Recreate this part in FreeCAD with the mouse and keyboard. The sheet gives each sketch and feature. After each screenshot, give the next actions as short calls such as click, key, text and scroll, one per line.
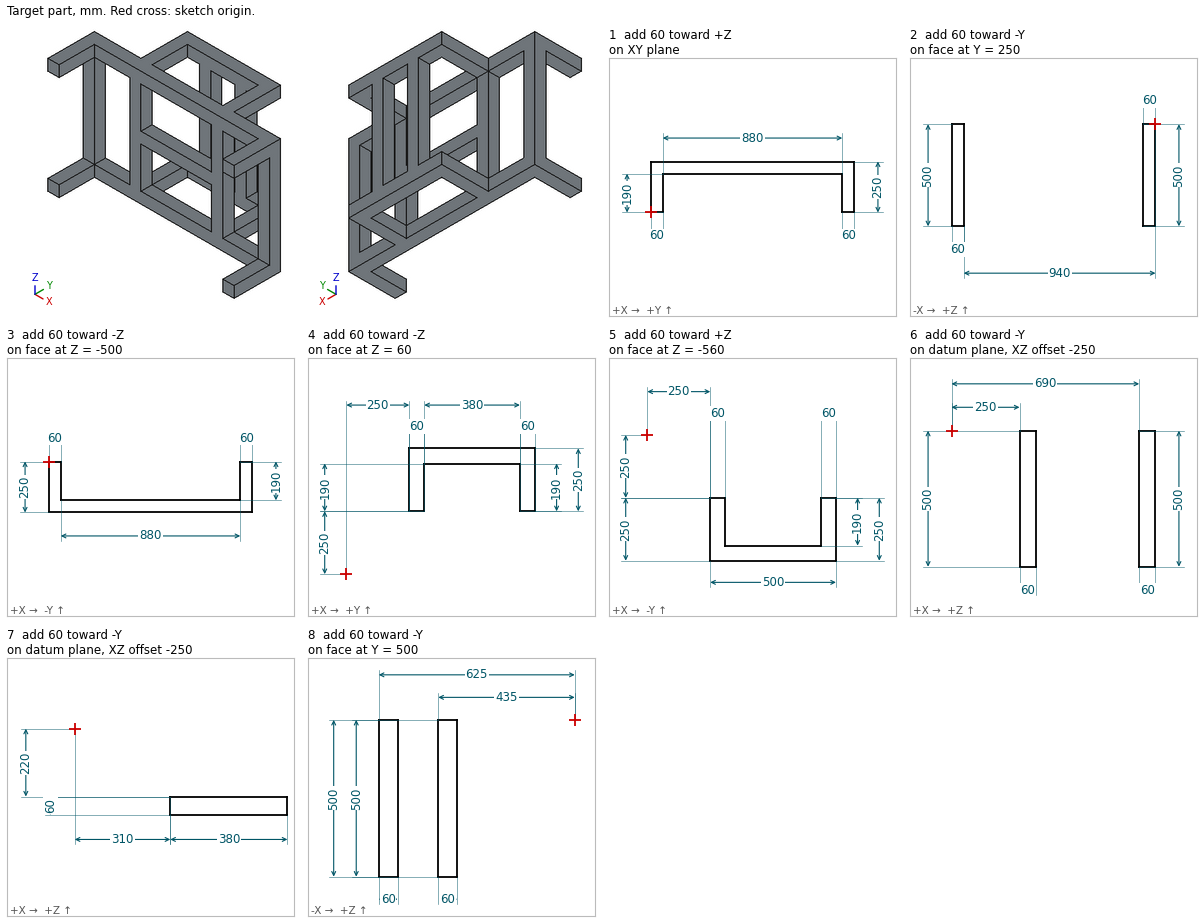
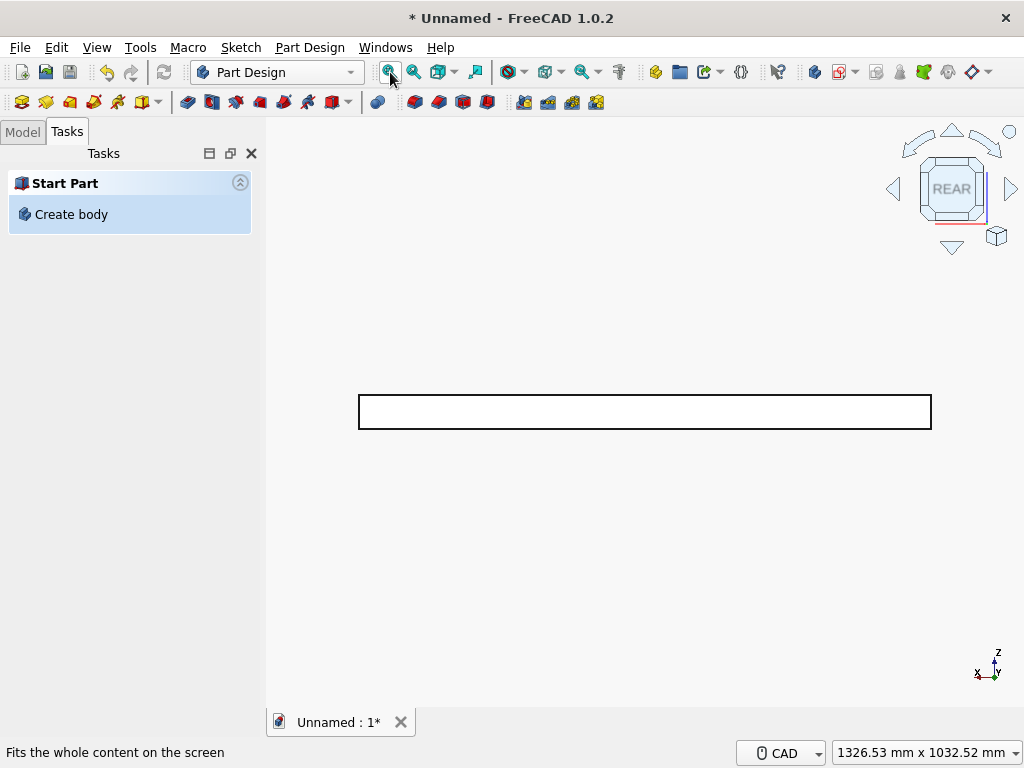
click(400, 411)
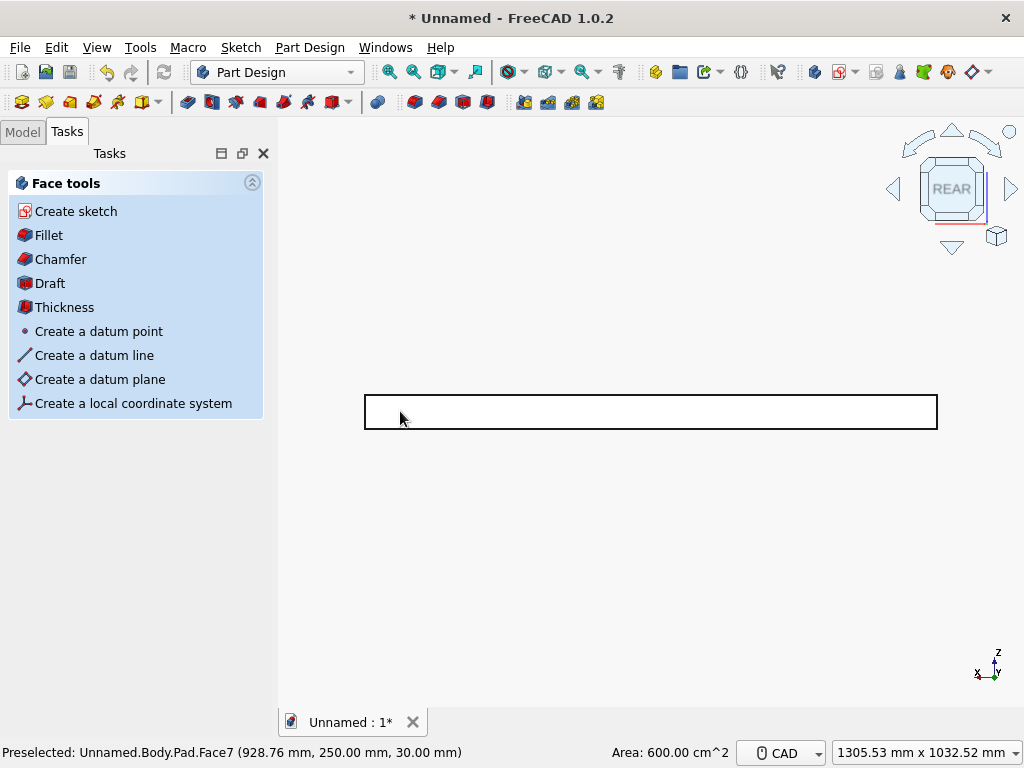
click(840, 72)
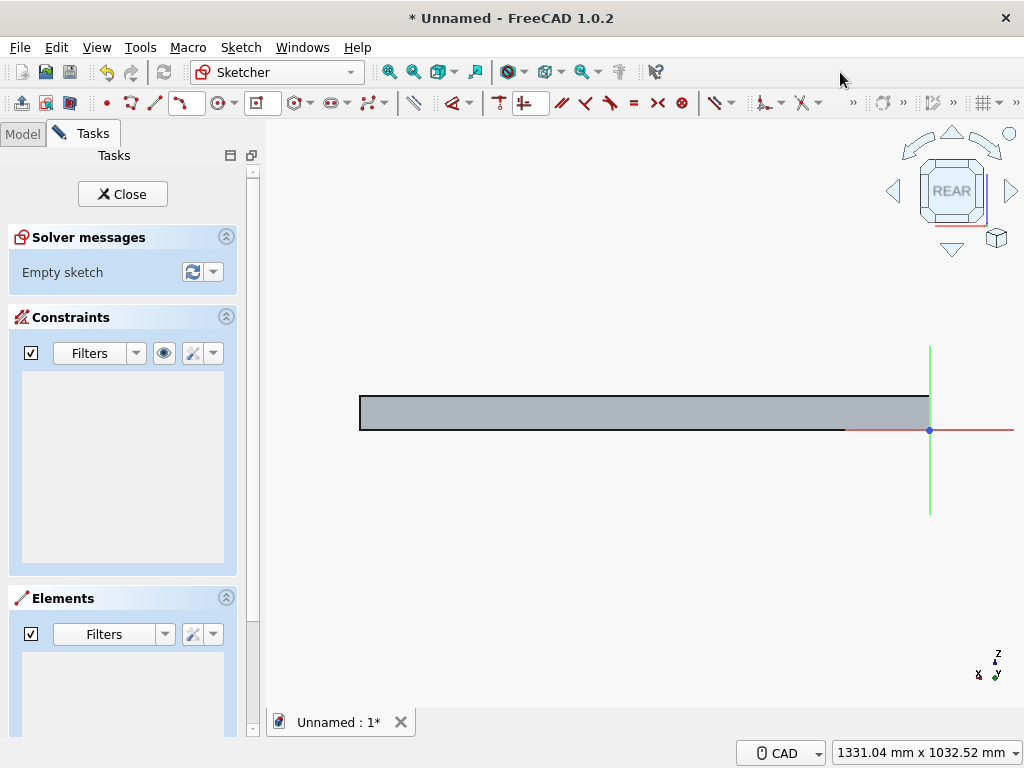
scroll(437, 147, down, 2)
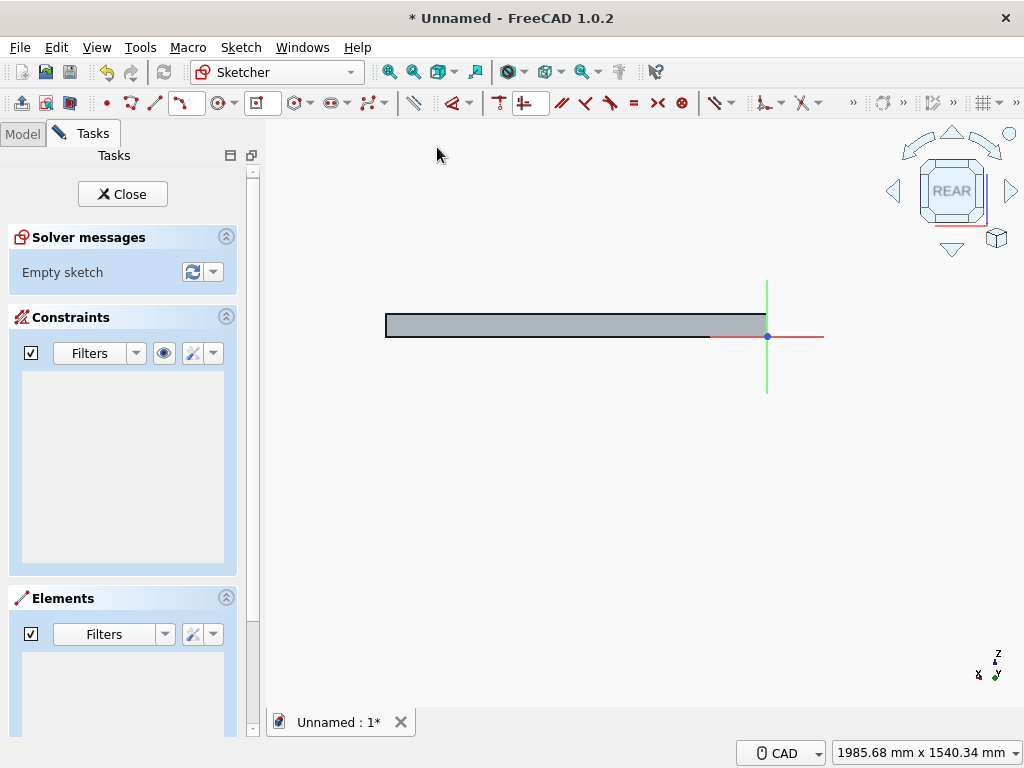
click(276, 104)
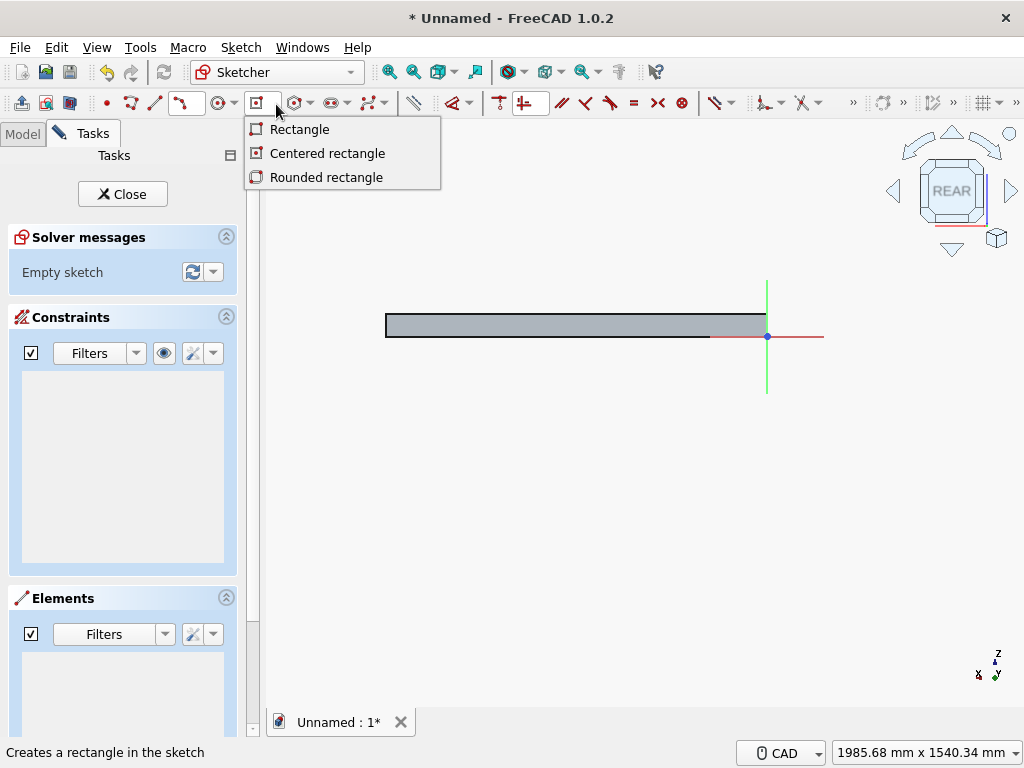
click(342, 129)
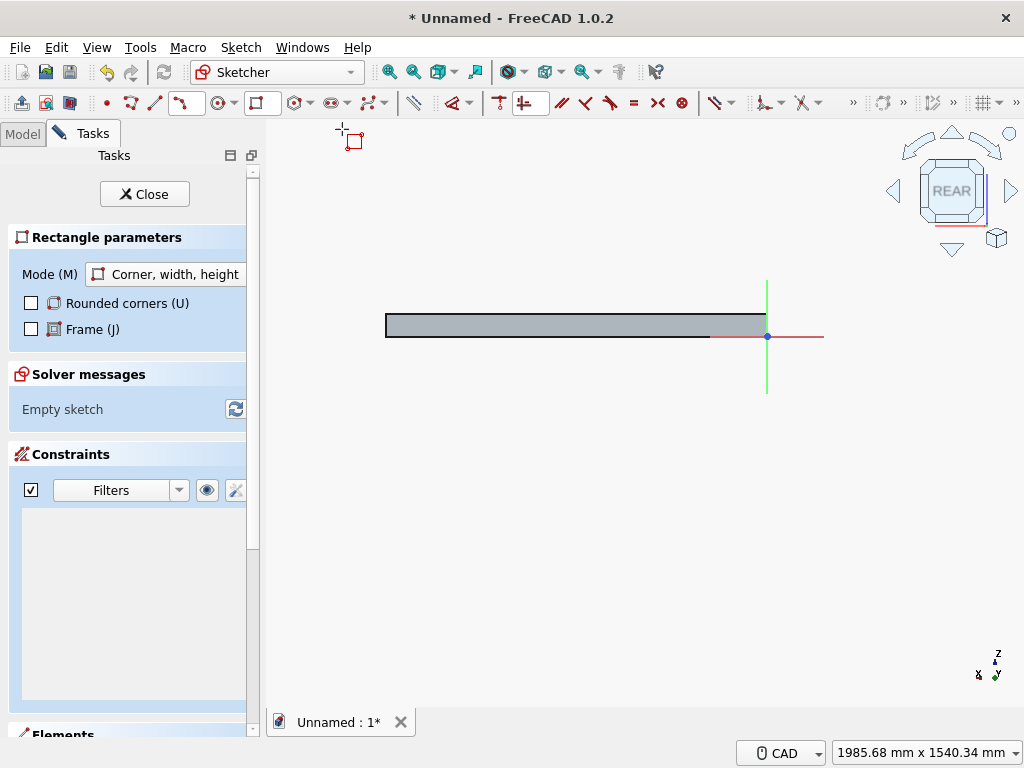
click(767, 337)
click(744, 528)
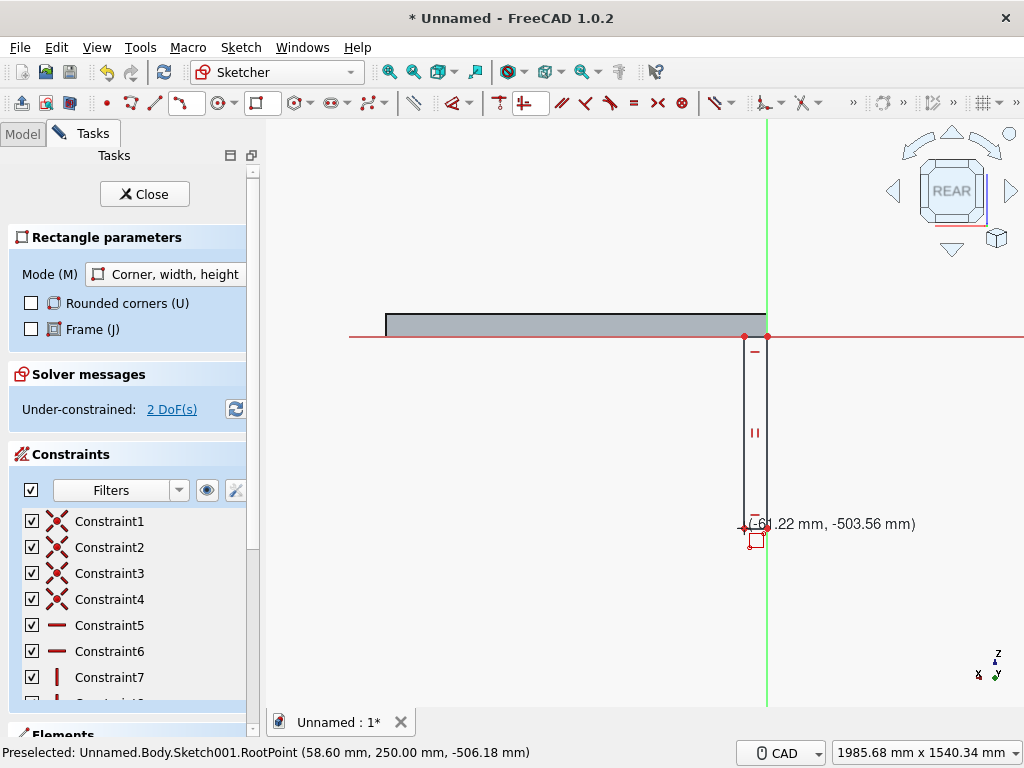
click(386, 337)
click(409, 528)
key(Escape)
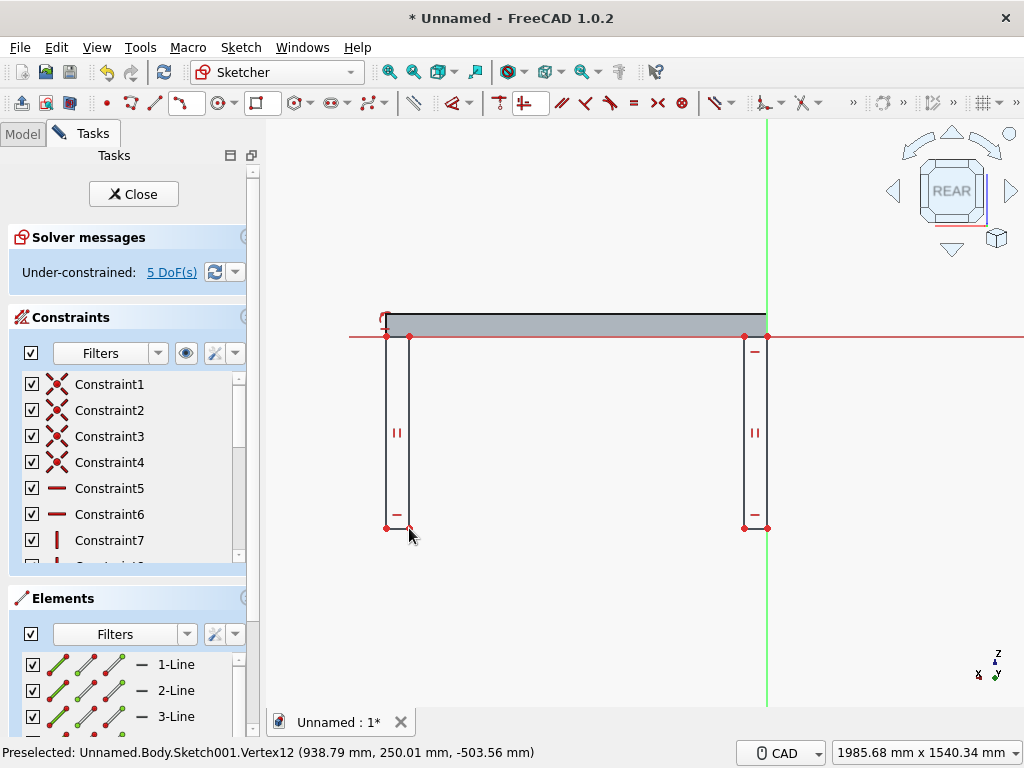
click(452, 104)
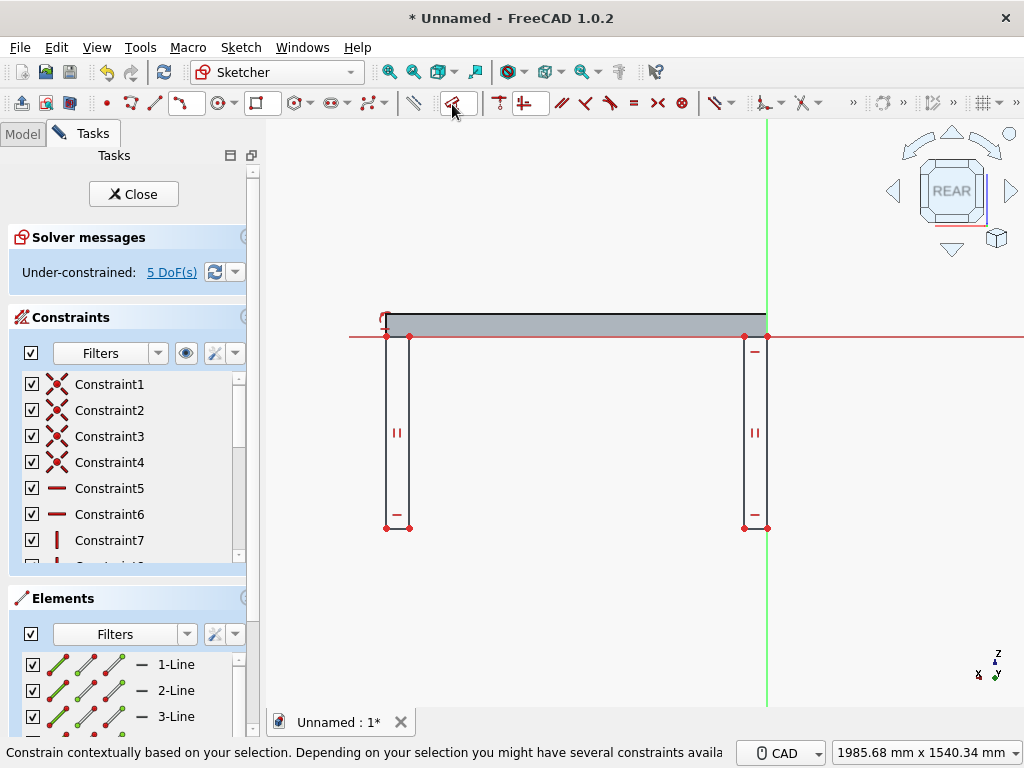
scroll(758, 337, up, 3)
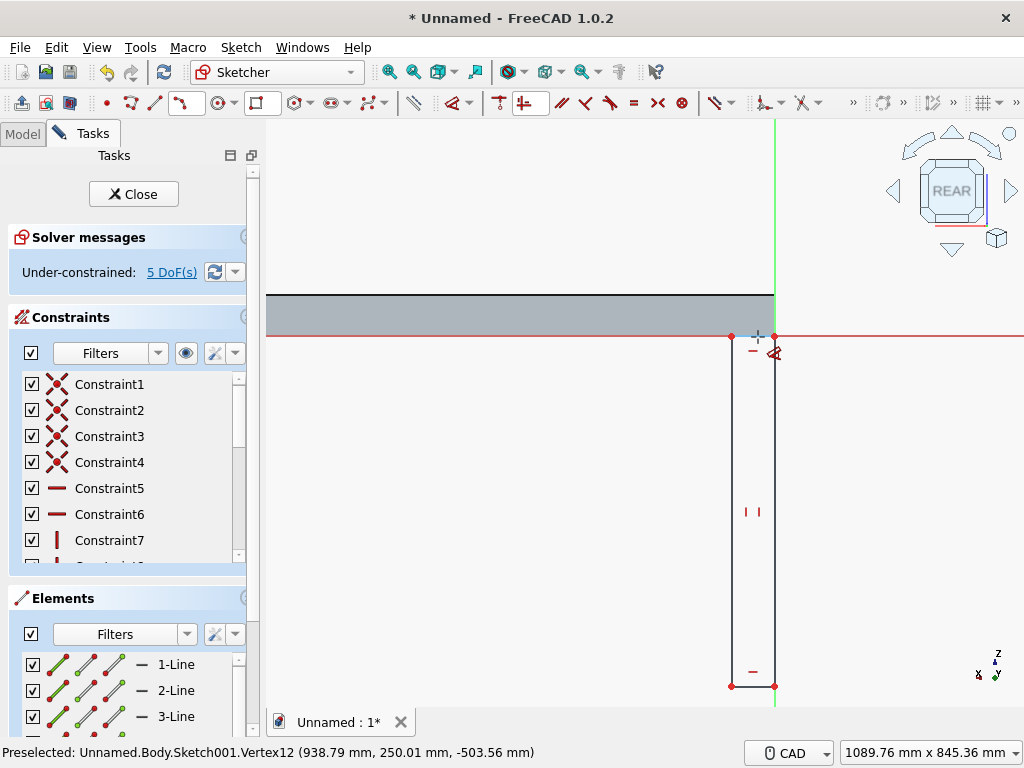
click(758, 336)
click(753, 302)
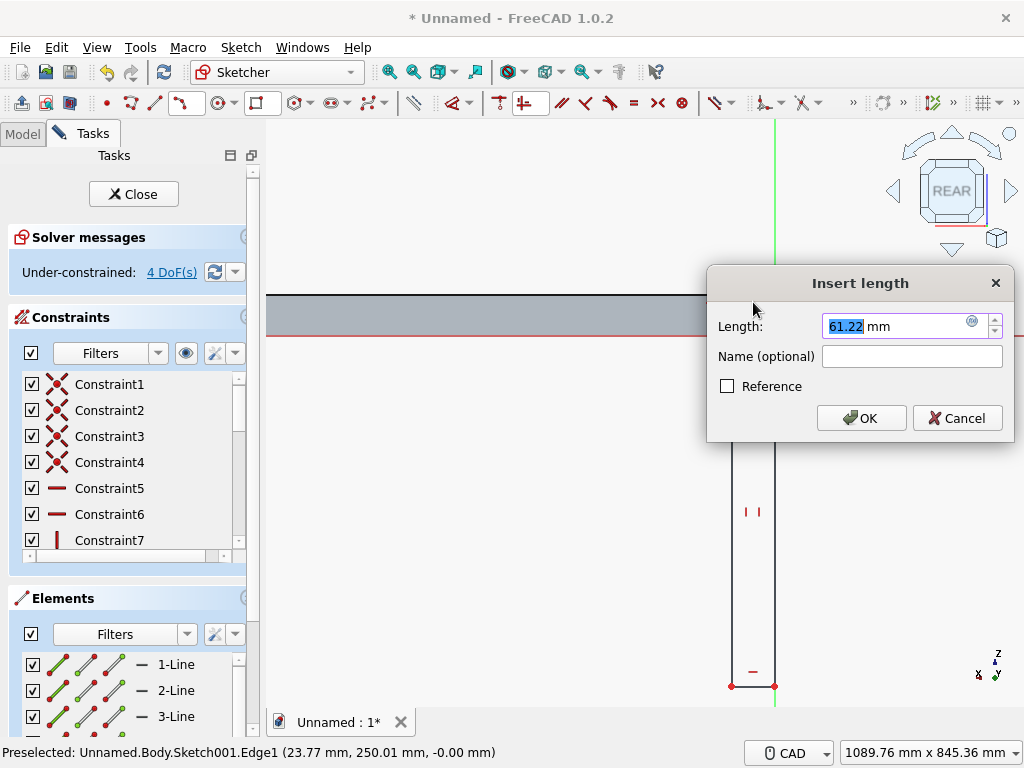
text(60)
key(Return)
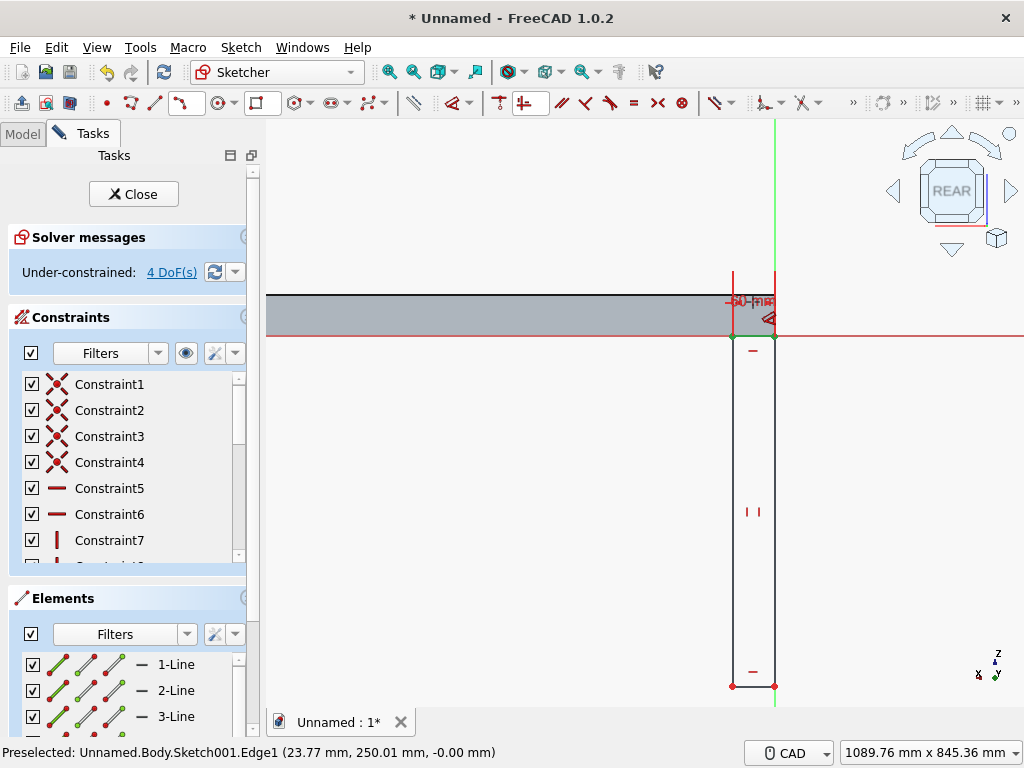
scroll(759, 295, down, 3)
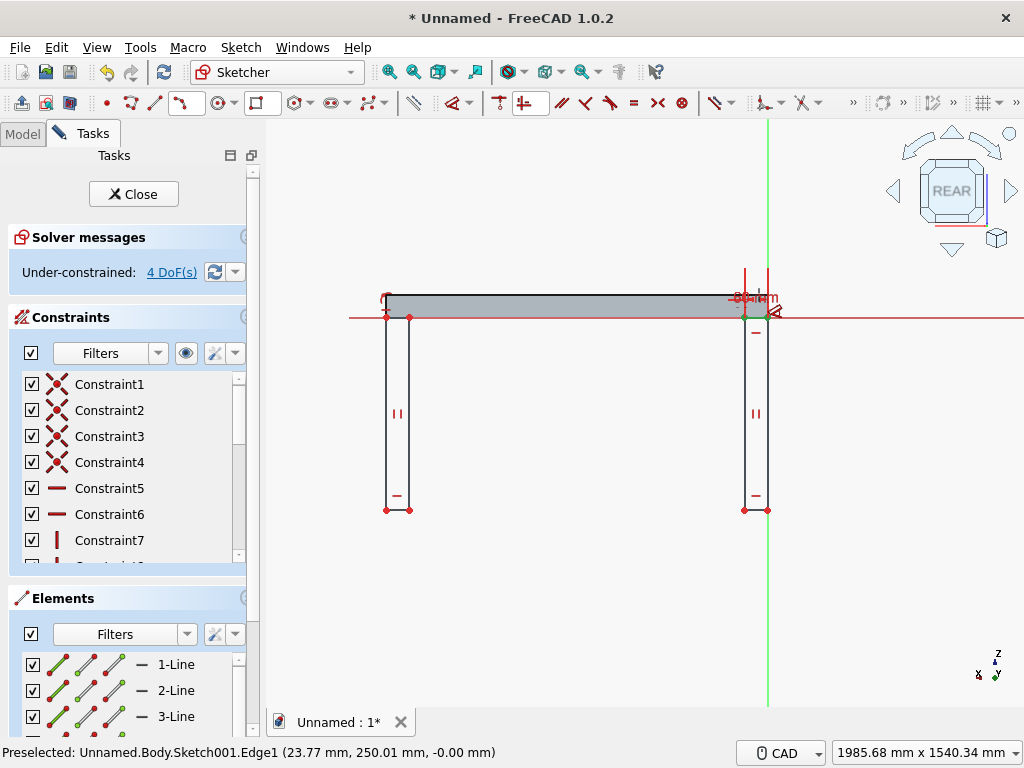
scroll(393, 510, up, 4)